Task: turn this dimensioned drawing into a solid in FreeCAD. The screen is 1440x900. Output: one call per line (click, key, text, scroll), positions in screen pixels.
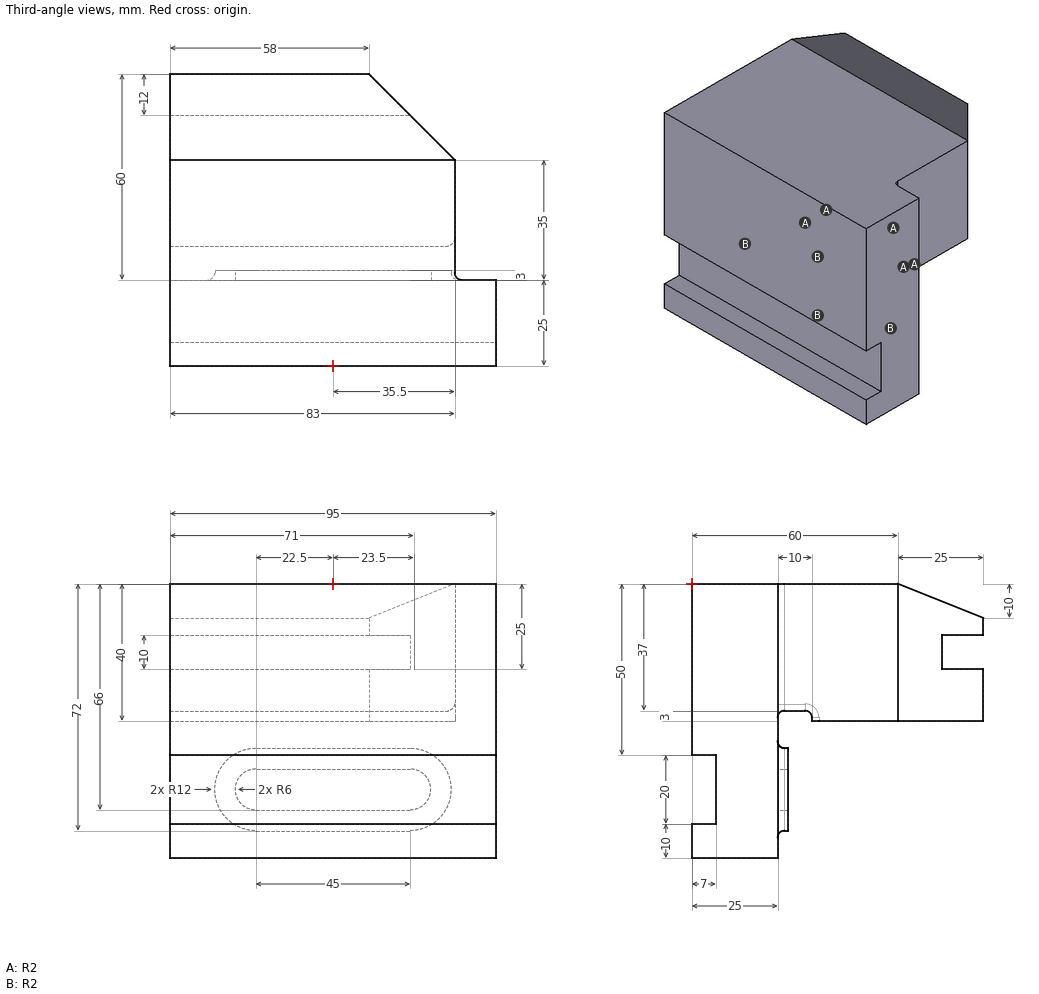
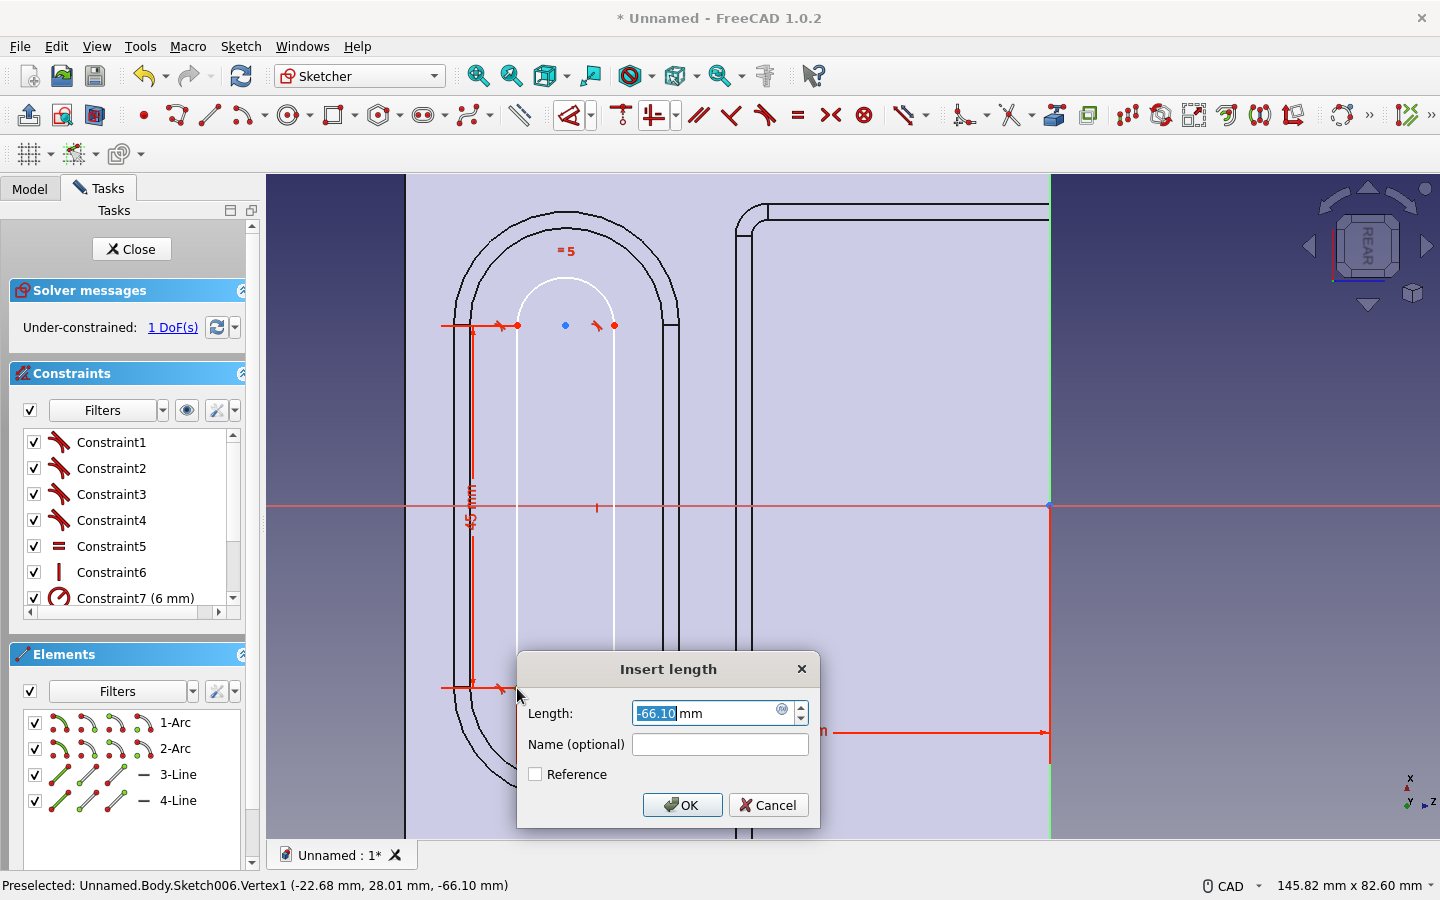
text(-66)
key(Return)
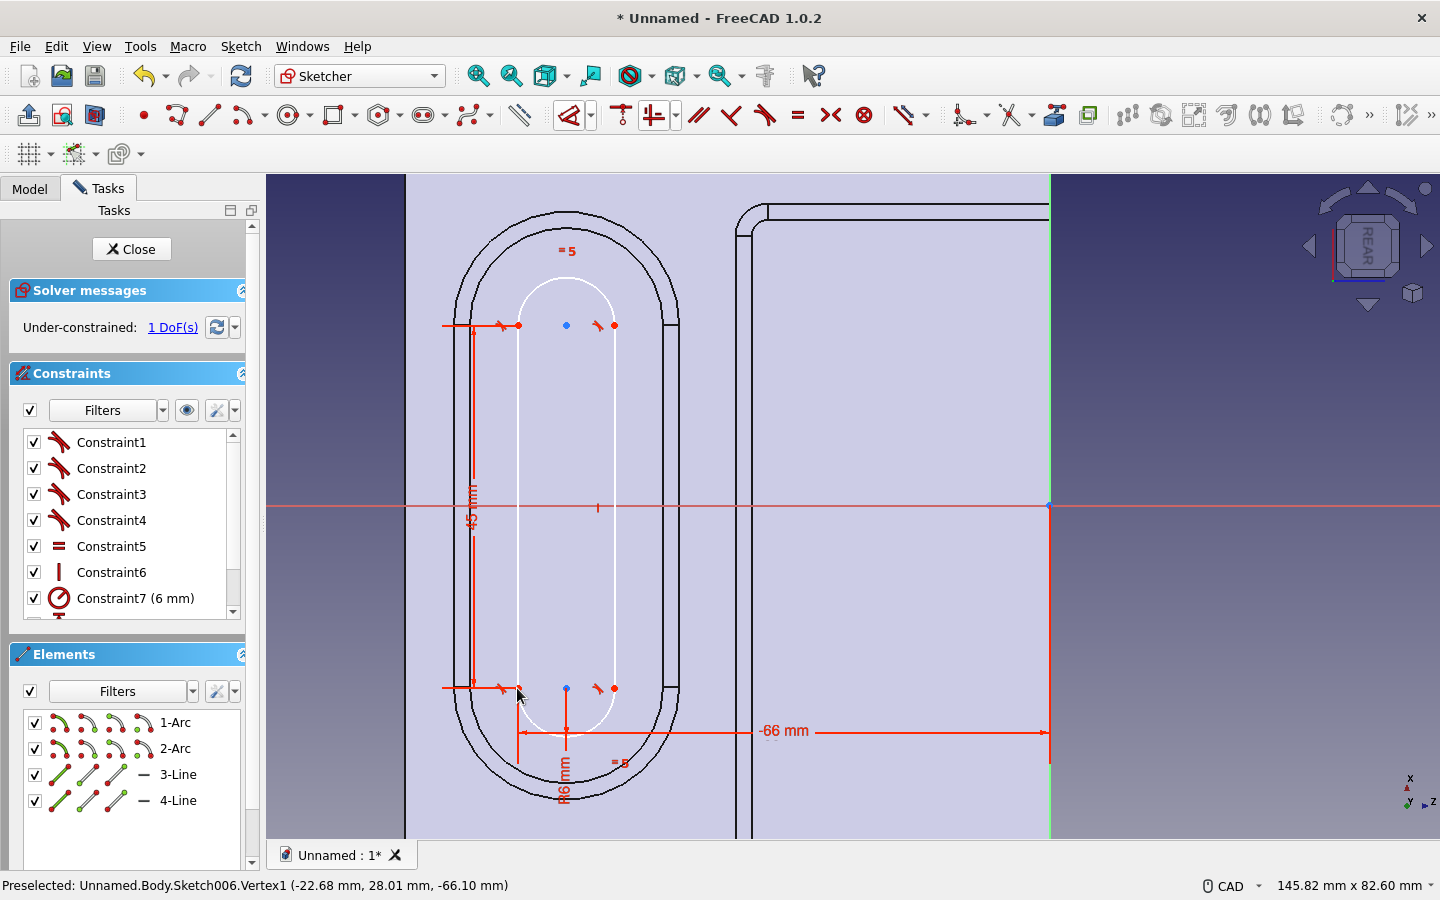
click(518, 688)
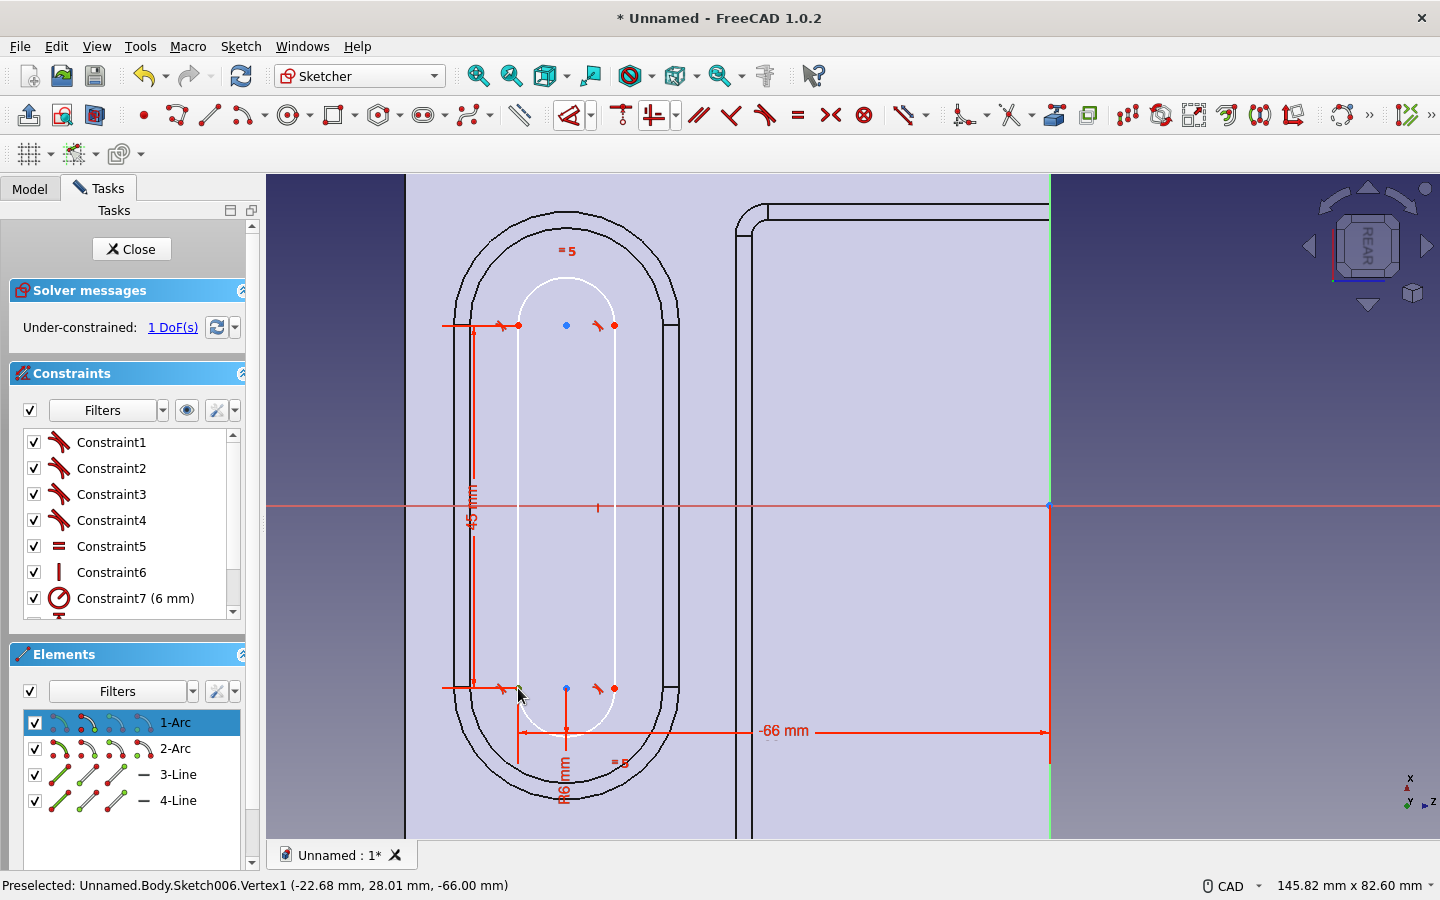
key(i)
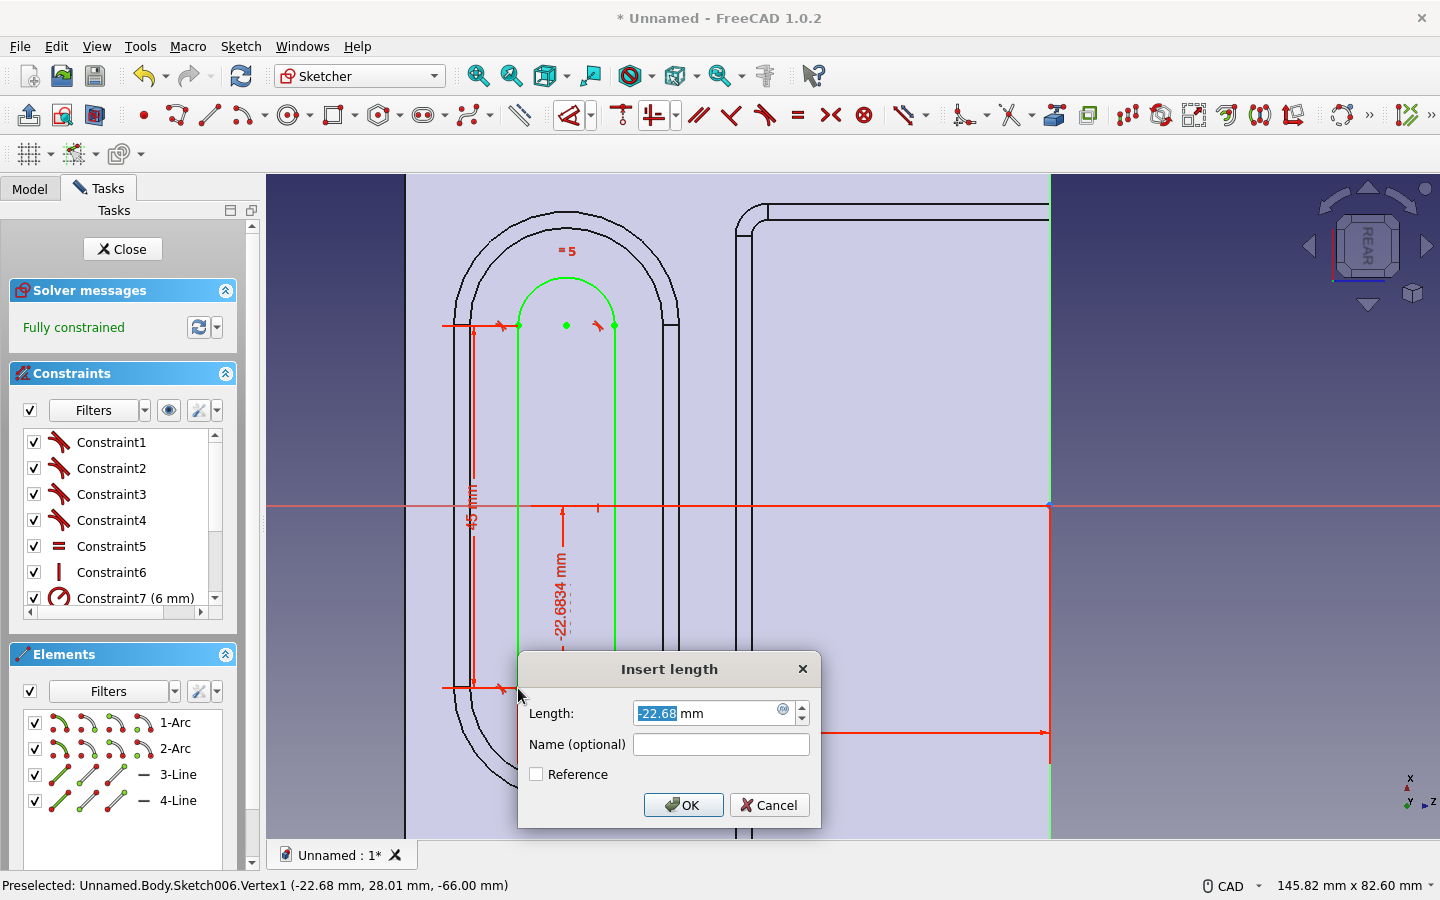
text(-22.5)
key(Return)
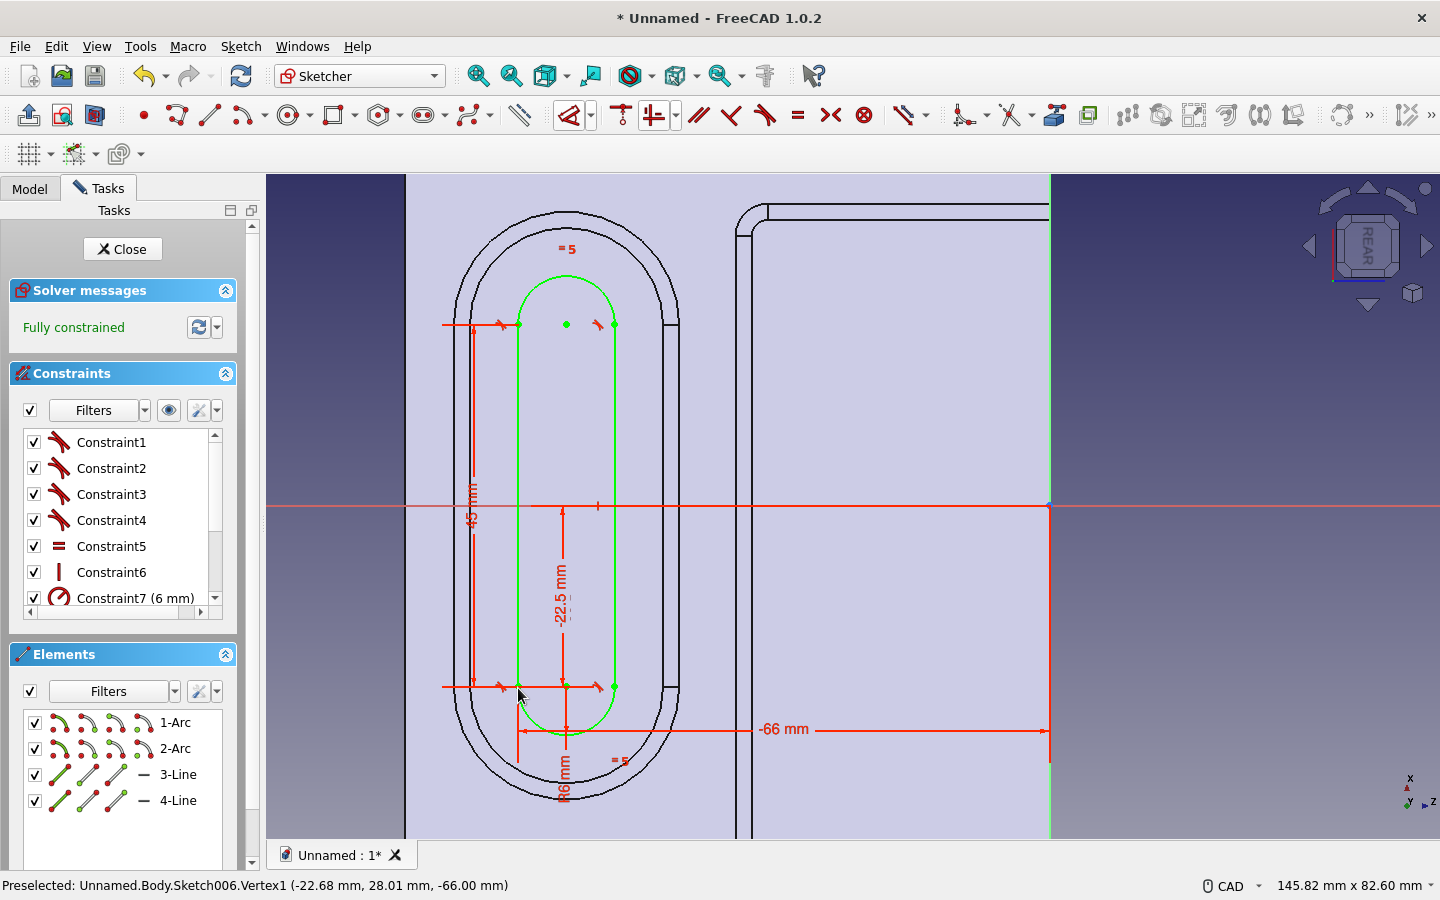
click(123, 249)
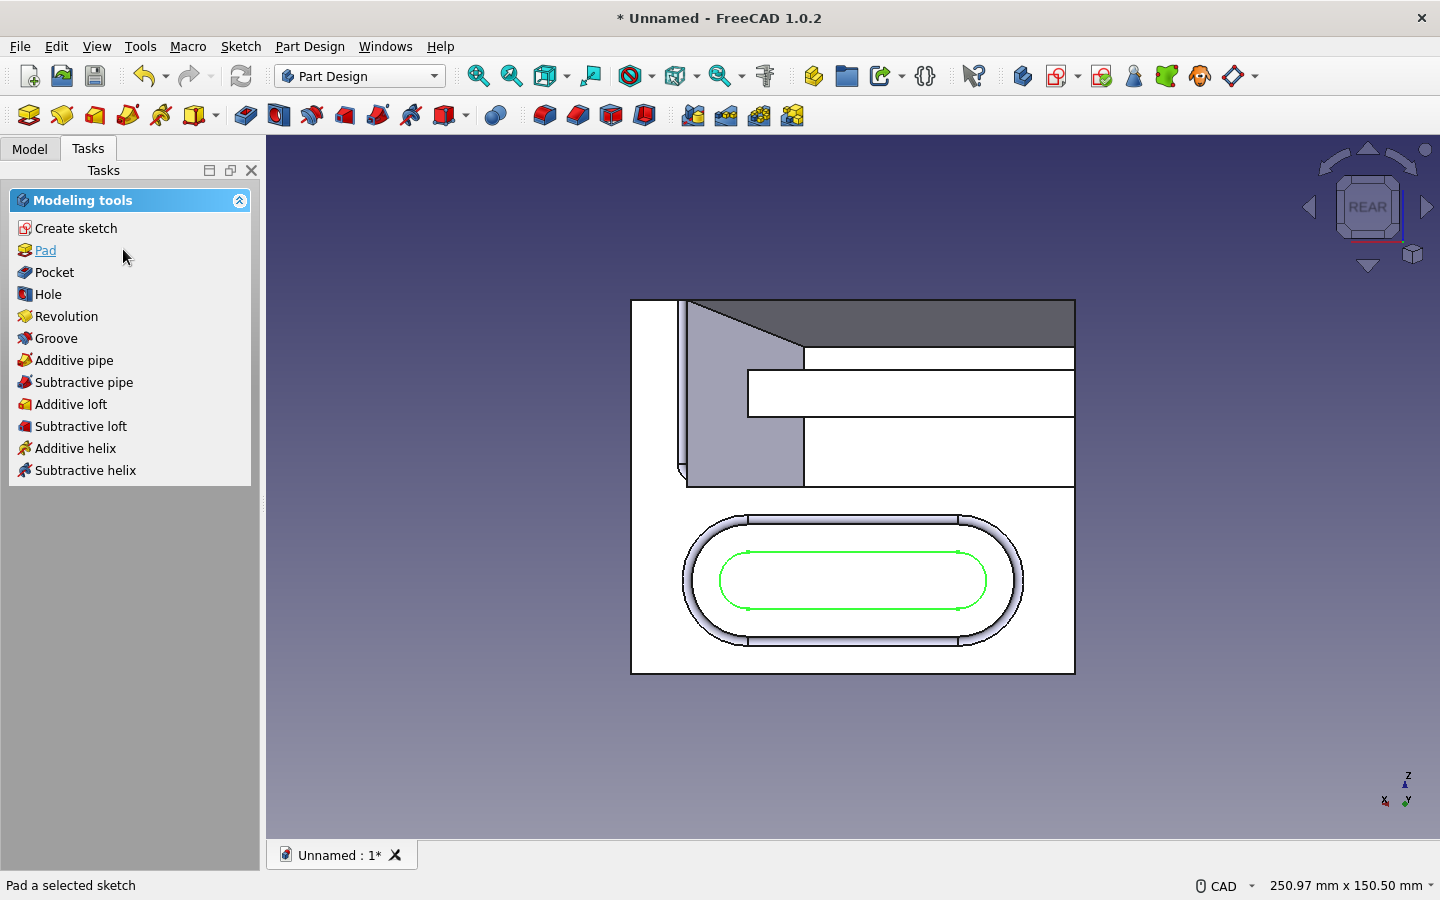
click(246, 116)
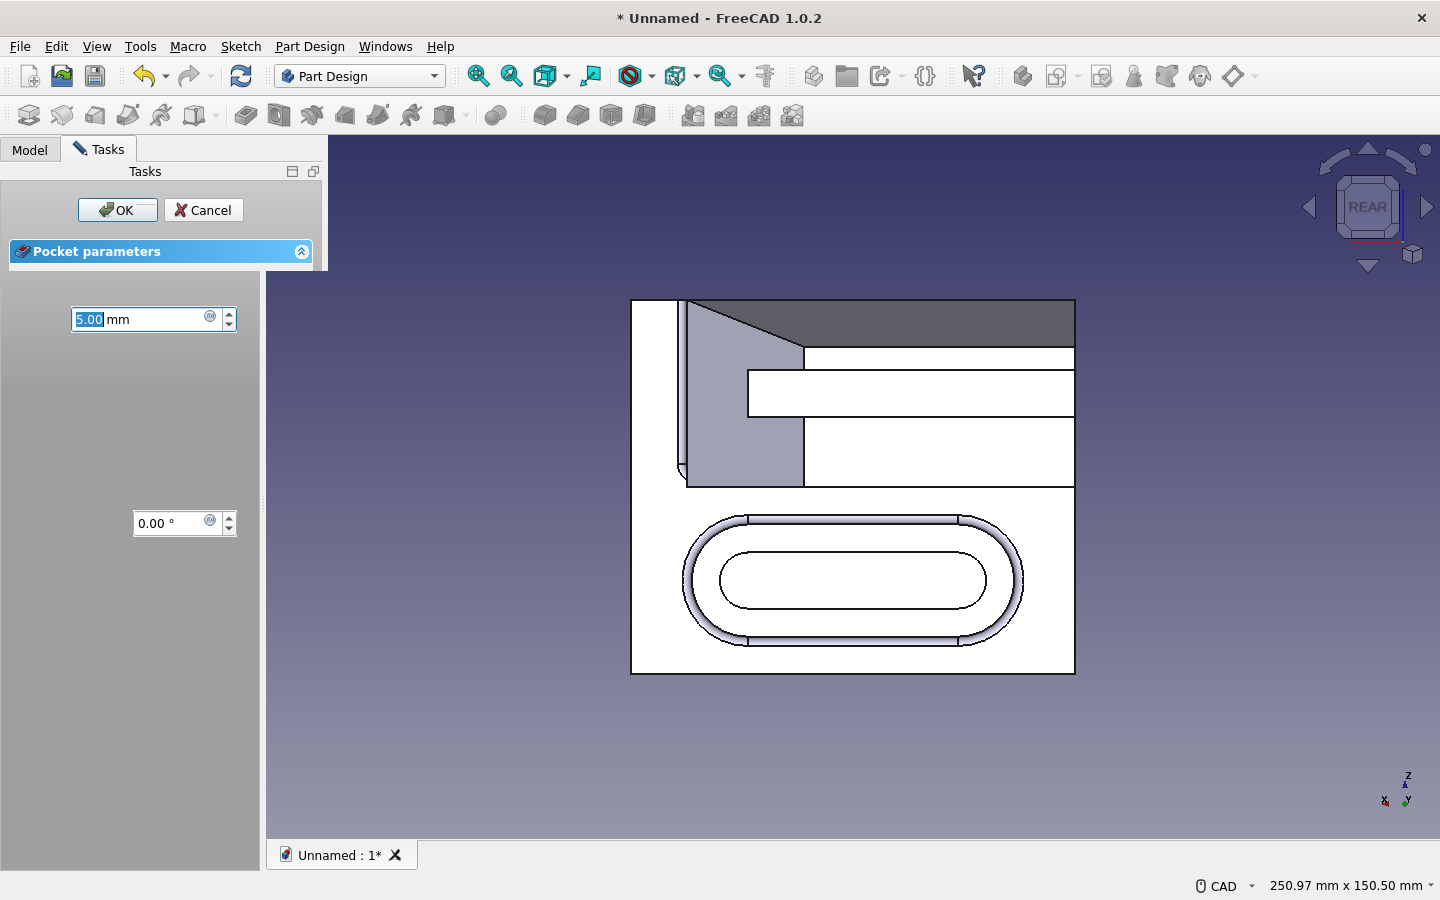
text(3)
key(Tab)